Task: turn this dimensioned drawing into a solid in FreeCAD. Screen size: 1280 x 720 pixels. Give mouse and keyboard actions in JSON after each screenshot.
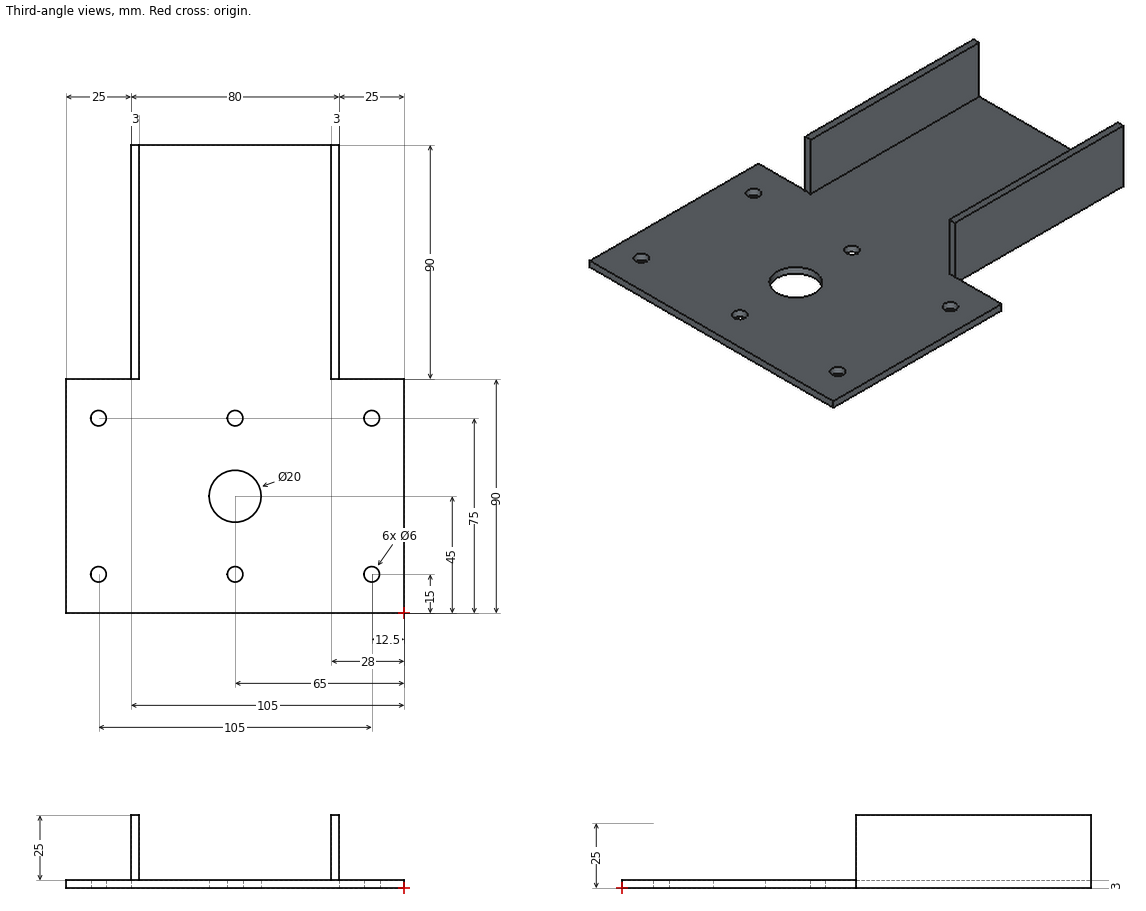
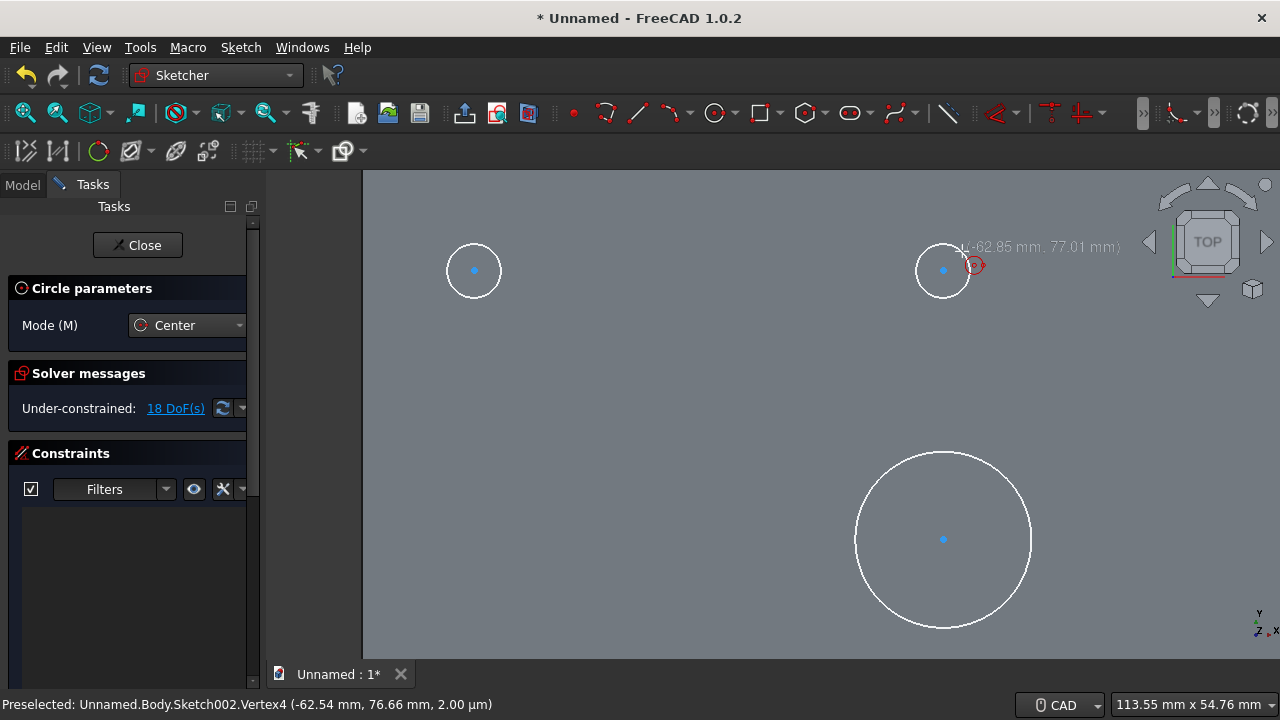
{"action": "scroll", "coordinate": [475, 270], "scroll_direction": "down", "scroll_amount": 4}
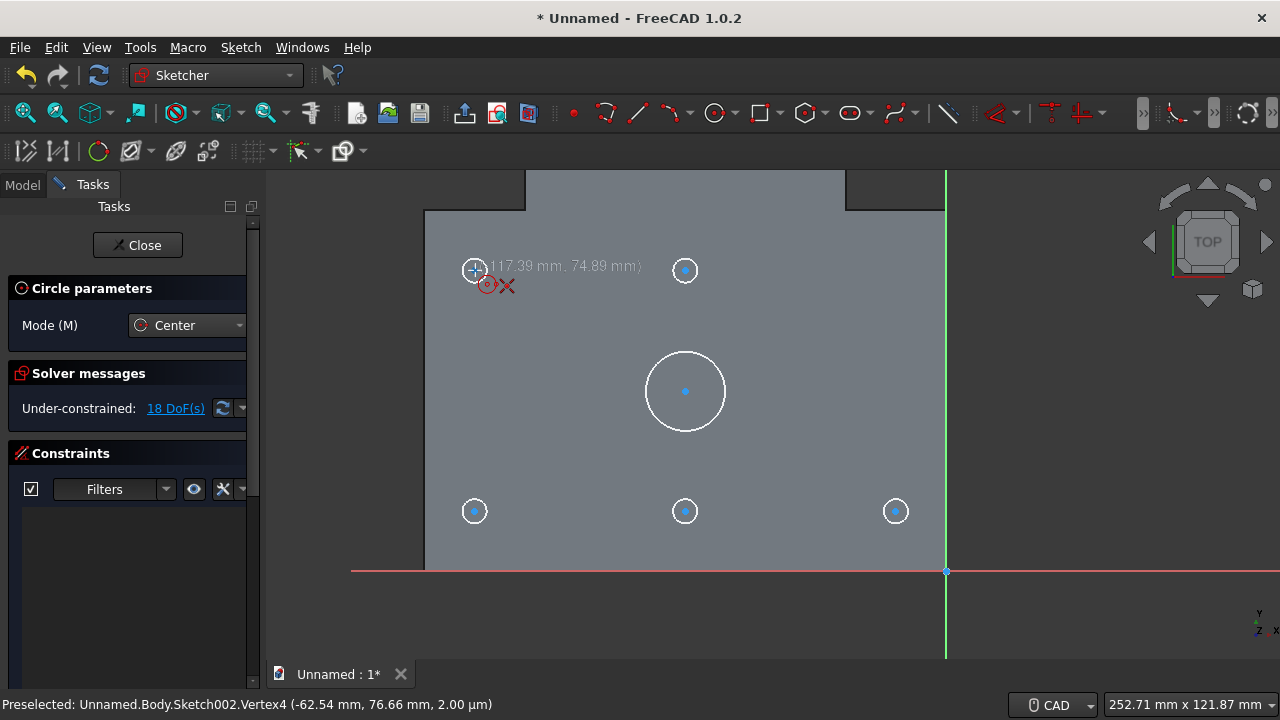
{"action": "scroll", "coordinate": [896, 270], "scroll_direction": "up", "scroll_amount": 4}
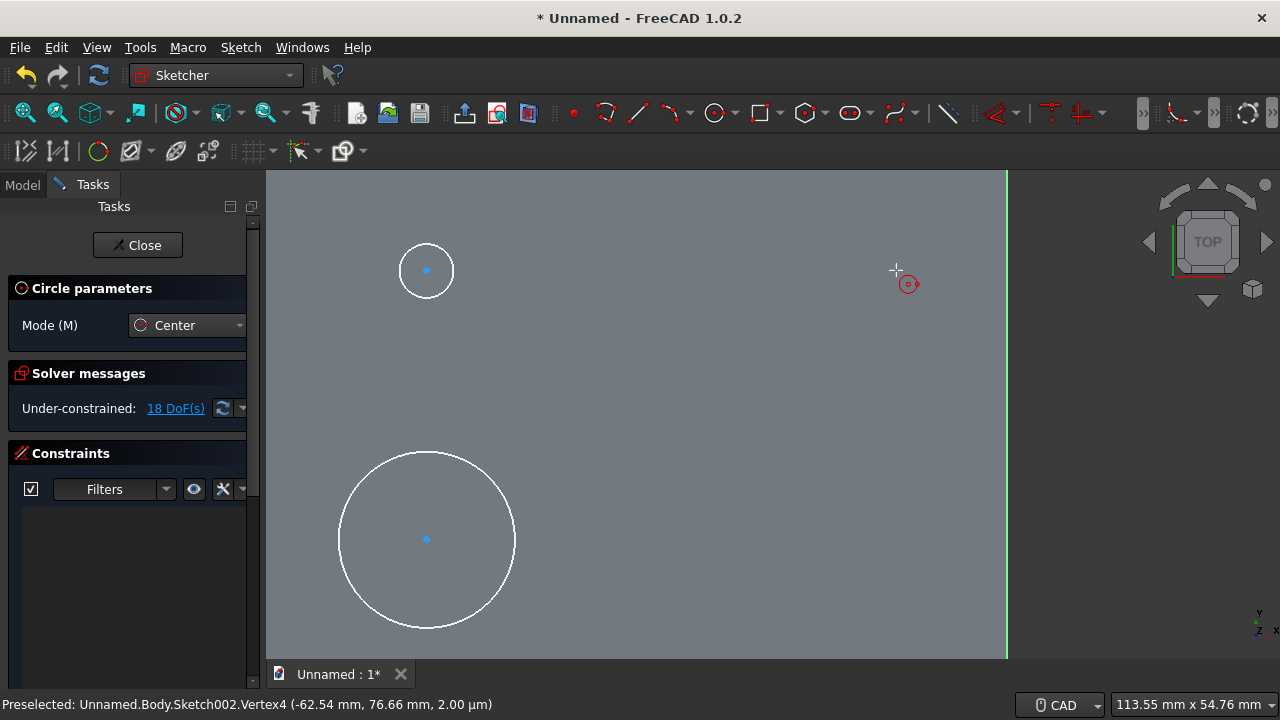
{"action": "left_click", "coordinate": [895, 270]}
{"action": "left_click", "coordinate": [914, 251]}
{"action": "key", "text": "Escape"}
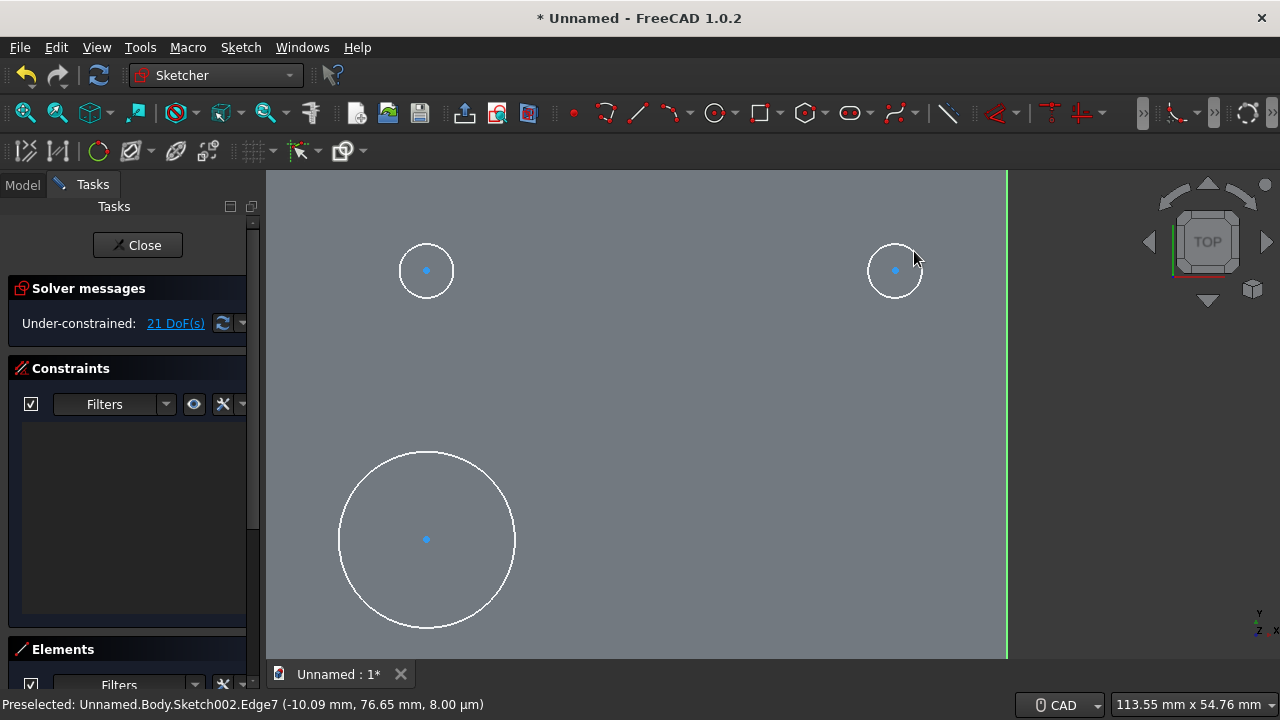
{"action": "scroll", "coordinate": [897, 270], "scroll_direction": "down", "scroll_amount": 4}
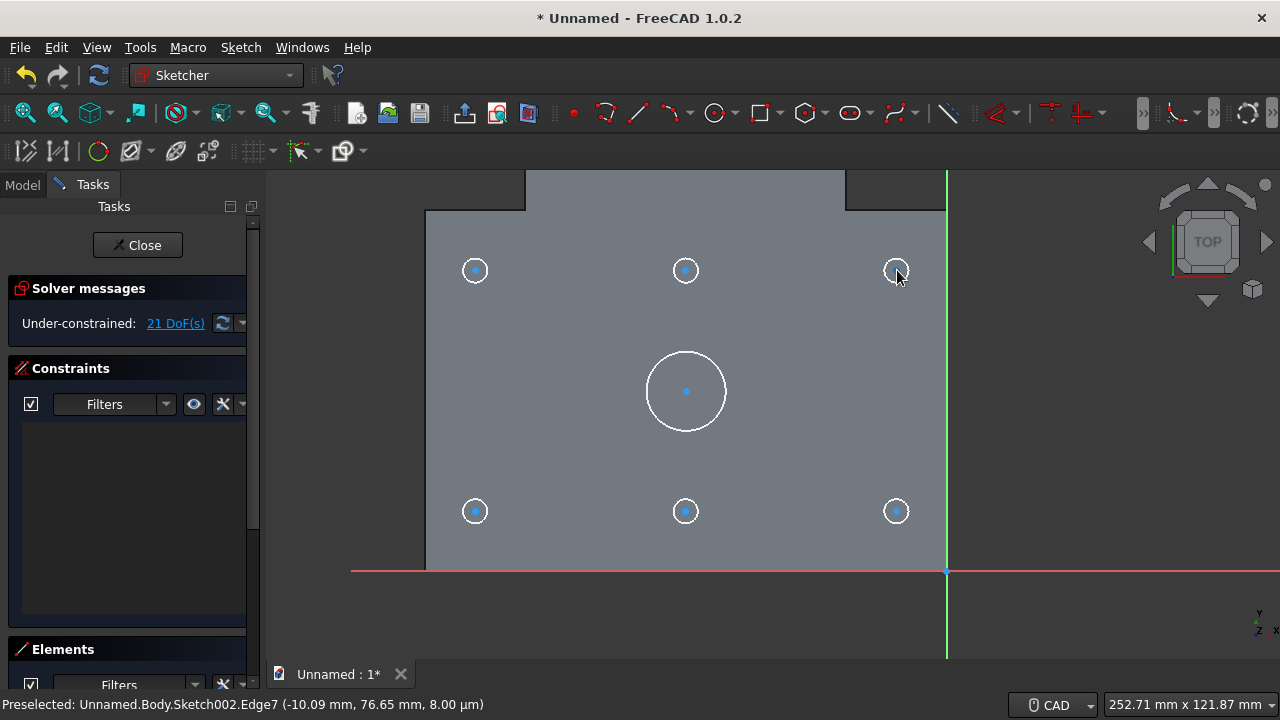
{"action": "left_click", "coordinate": [905, 503]}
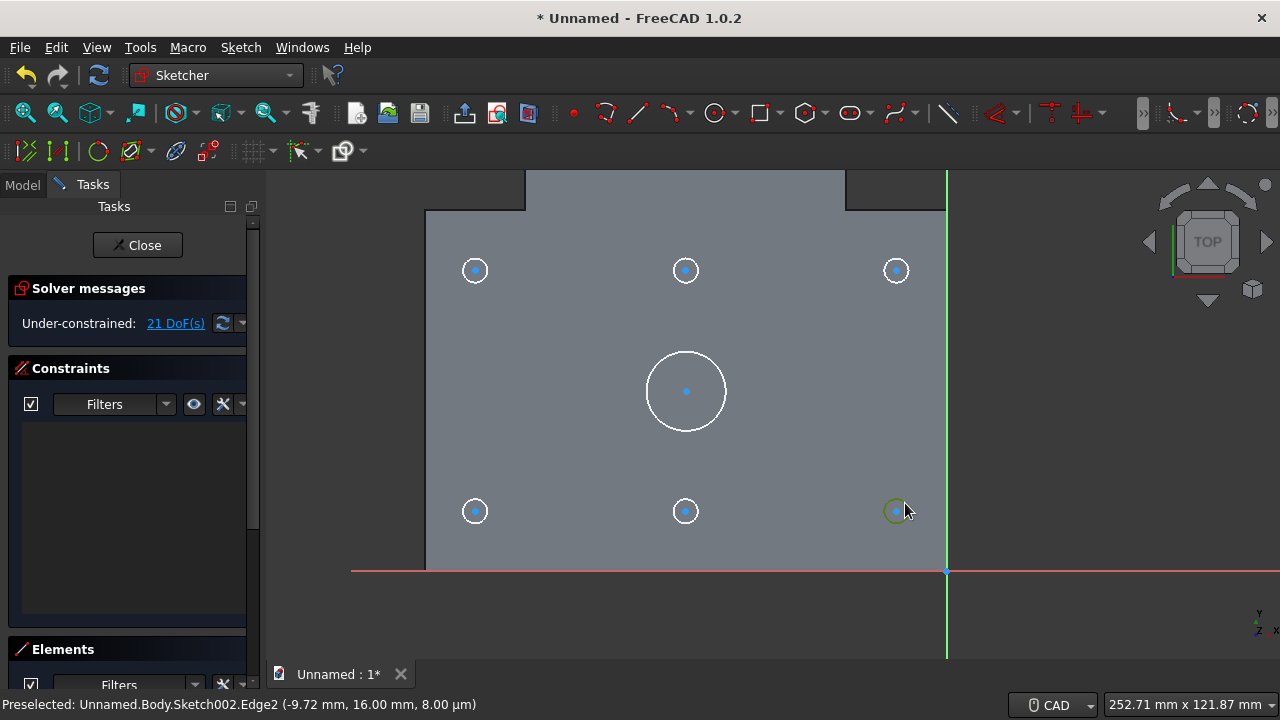
{"action": "left_click", "coordinate": [694, 503]}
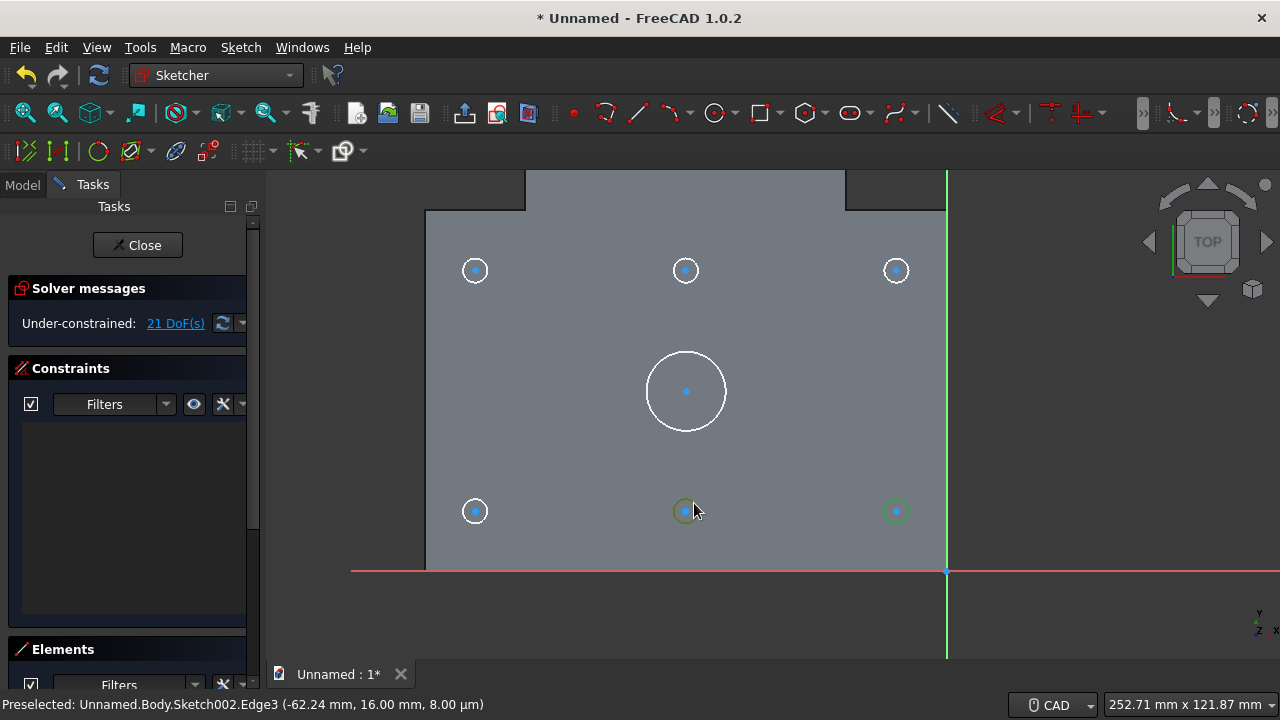
{"action": "left_click", "coordinate": [484, 503]}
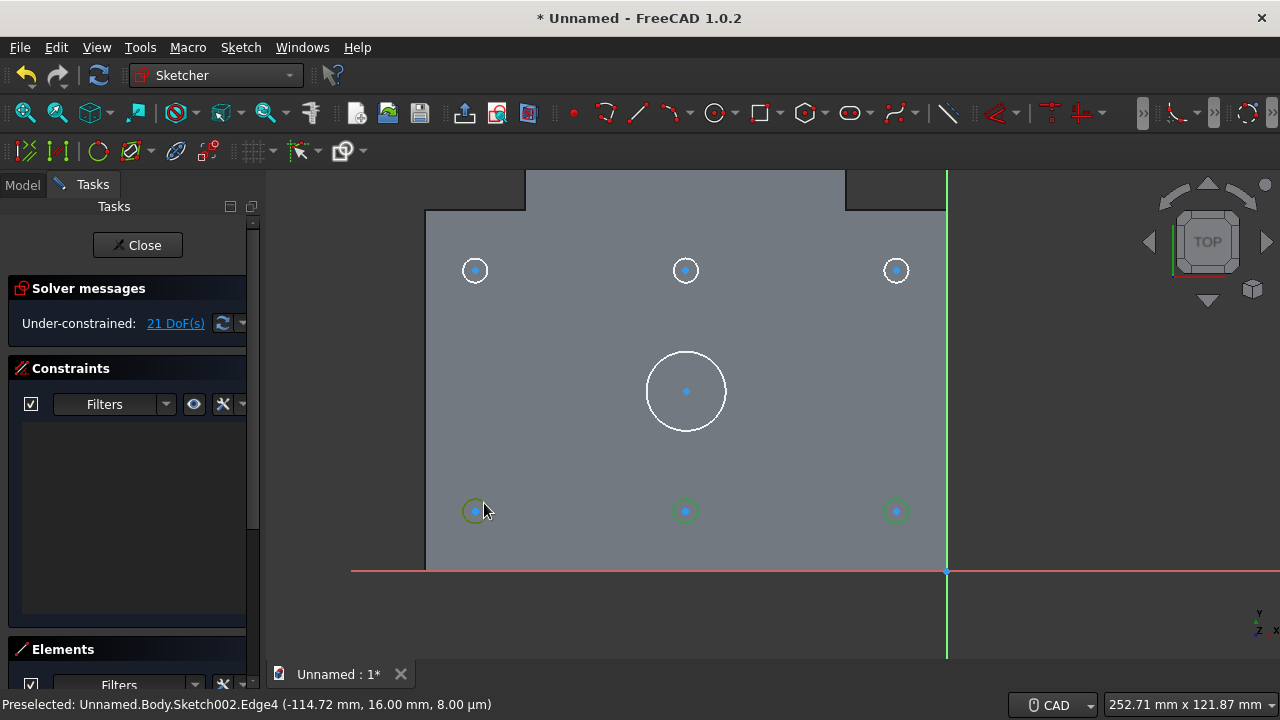
{"action": "left_click", "coordinate": [484, 262]}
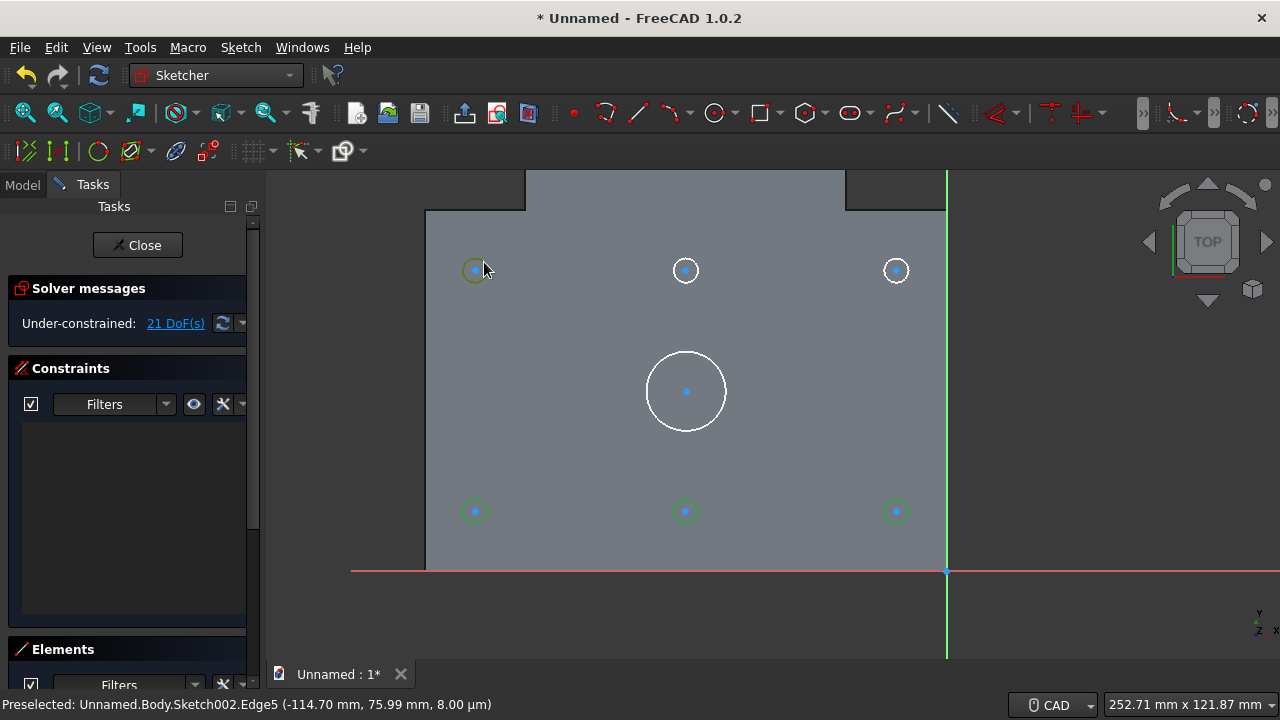
{"action": "left_click", "coordinate": [694, 262]}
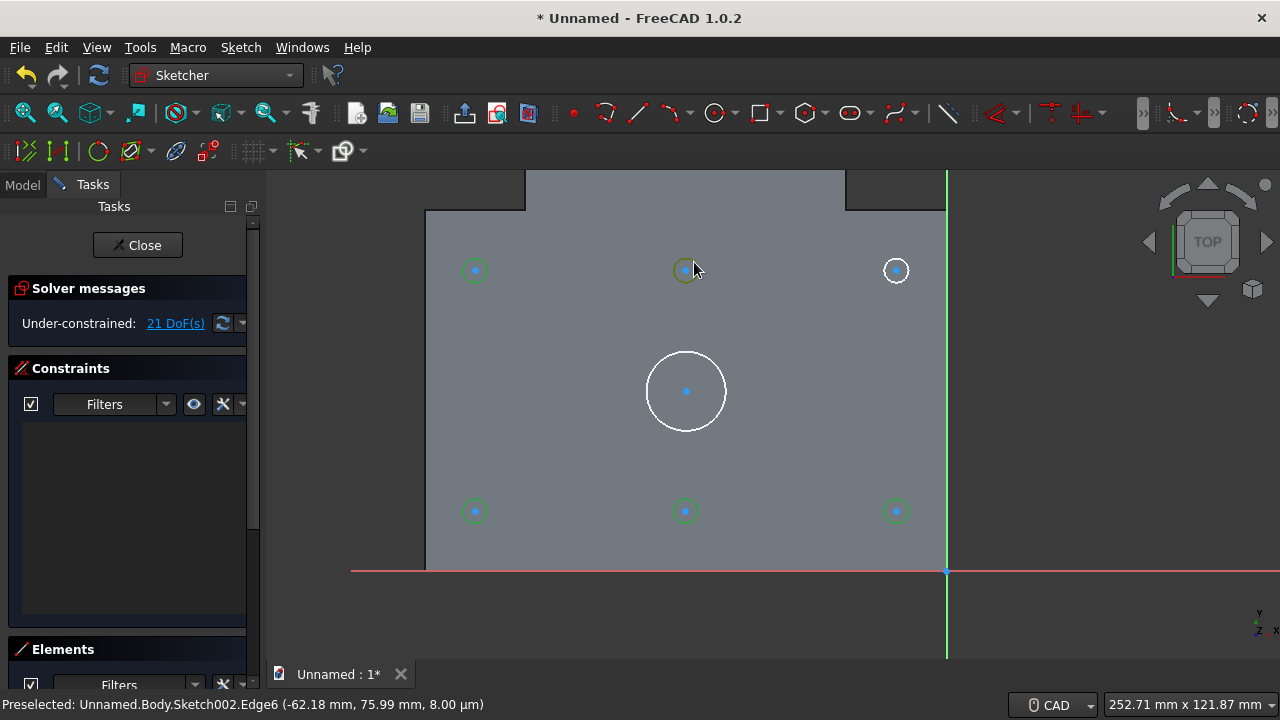
{"action": "left_click", "coordinate": [905, 262]}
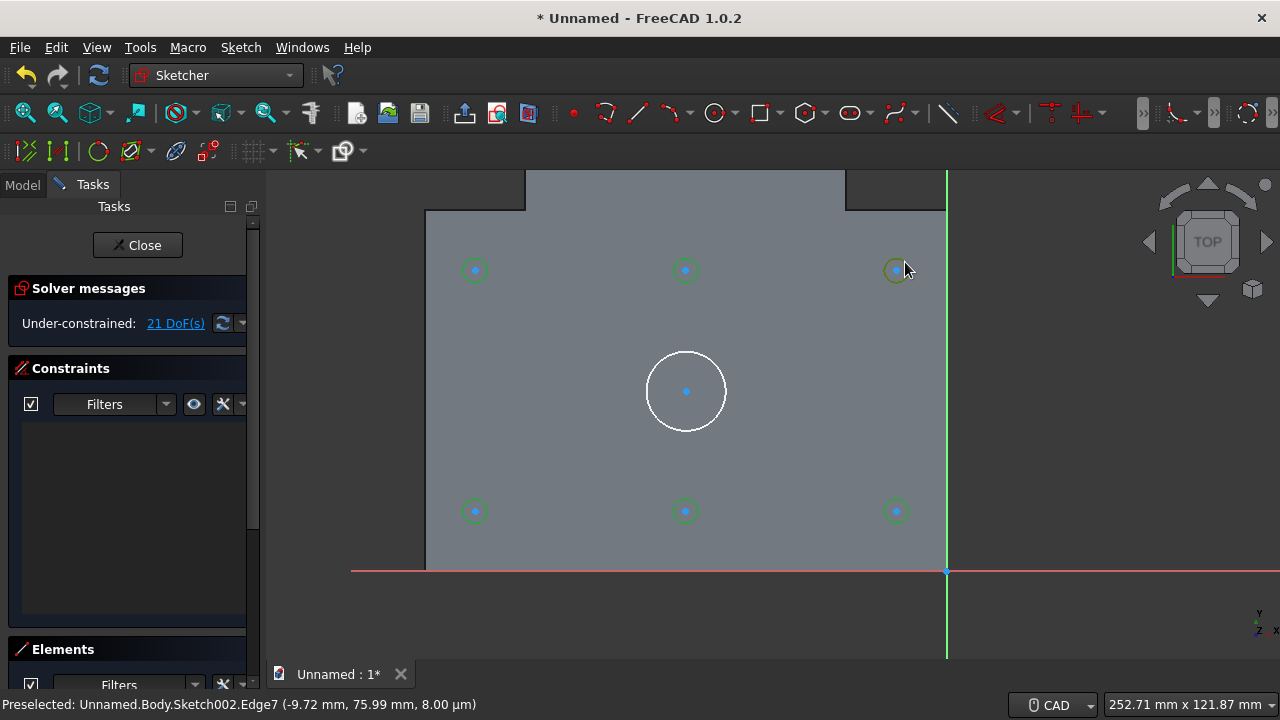
{"action": "key", "text": "e"}